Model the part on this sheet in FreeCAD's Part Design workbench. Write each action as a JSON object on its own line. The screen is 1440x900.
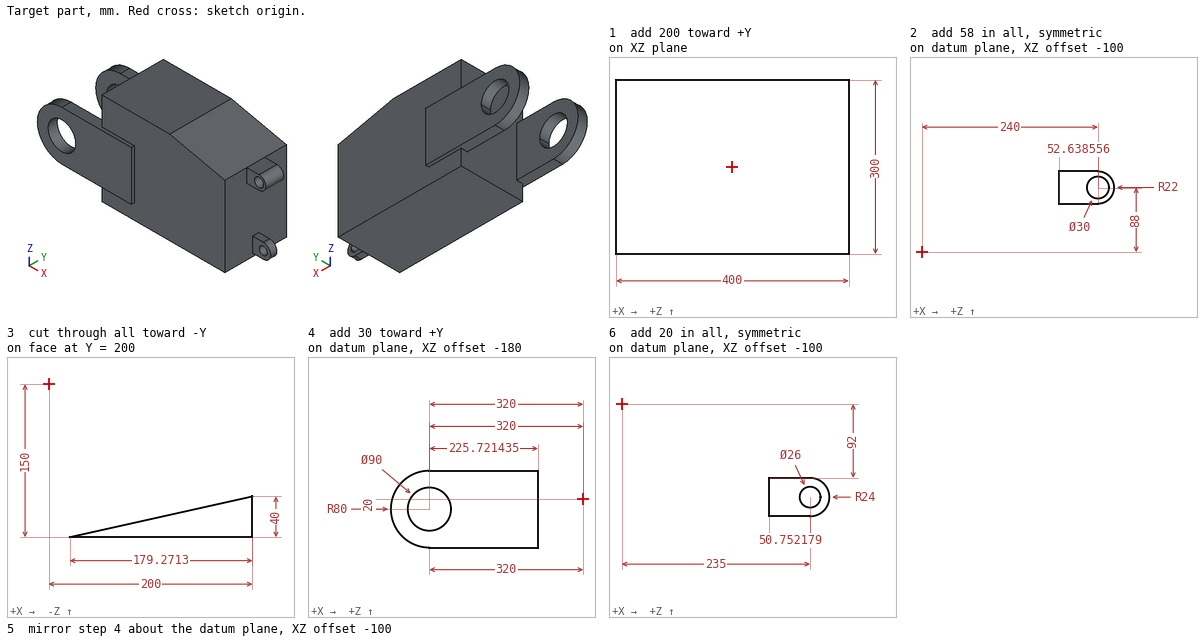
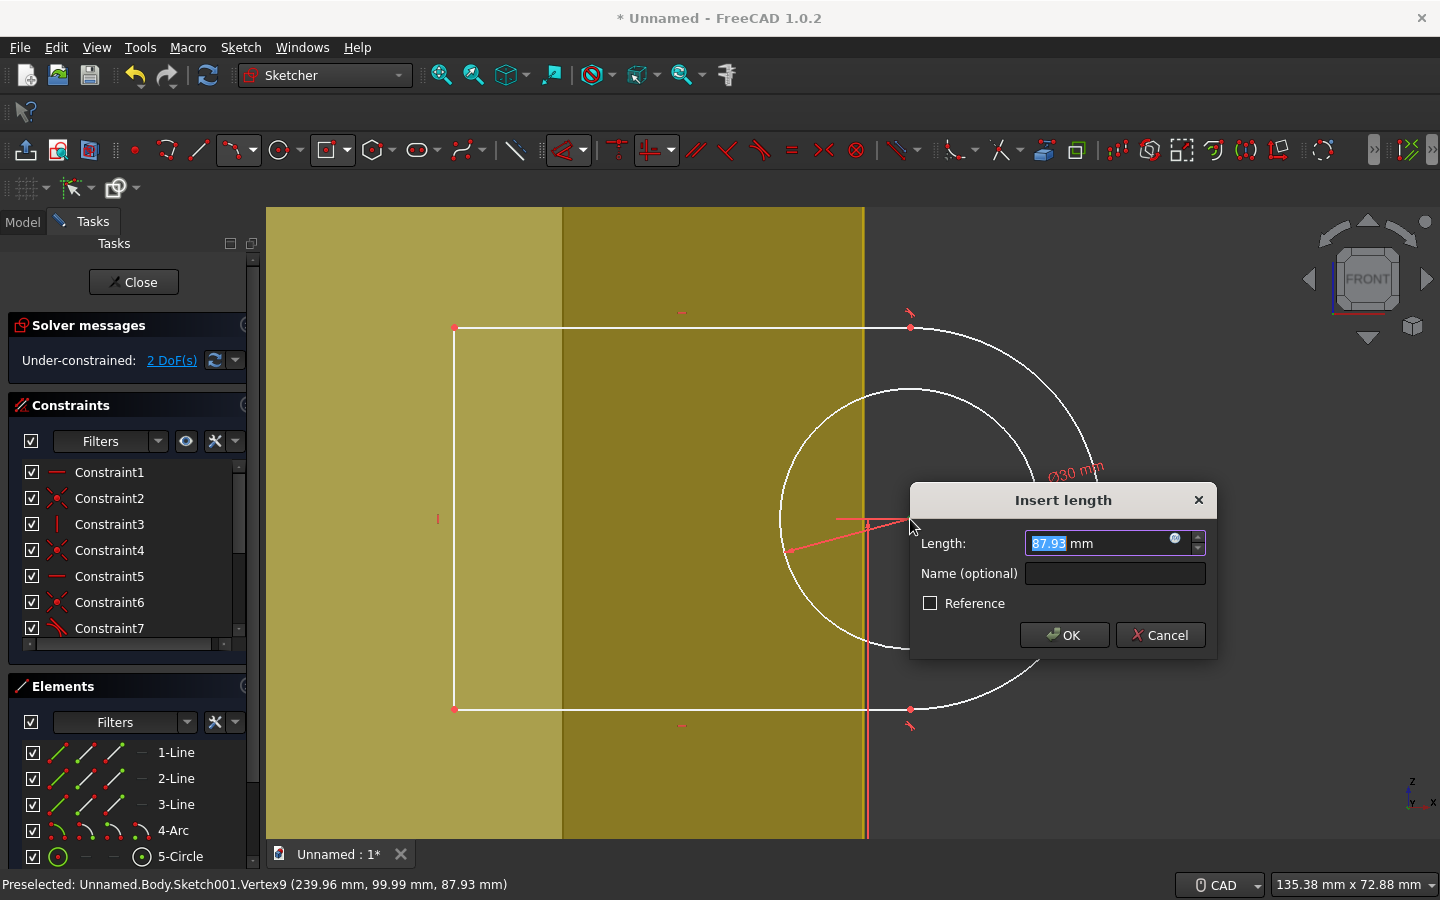
{"action": "type", "text": "88"}
{"action": "key", "text": "Return"}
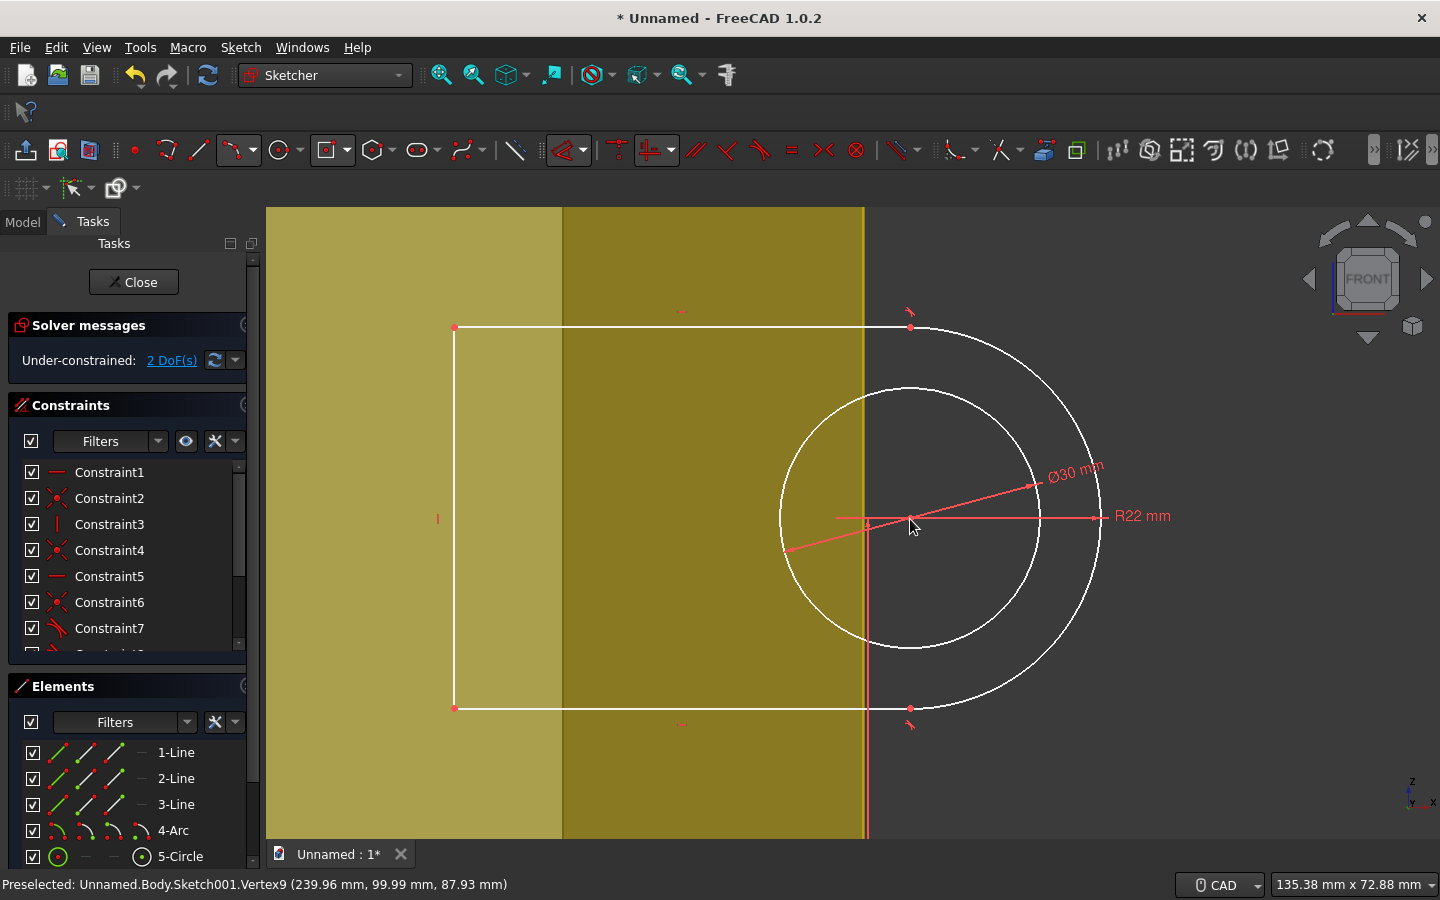
{"action": "left_click", "coordinate": [910, 518]}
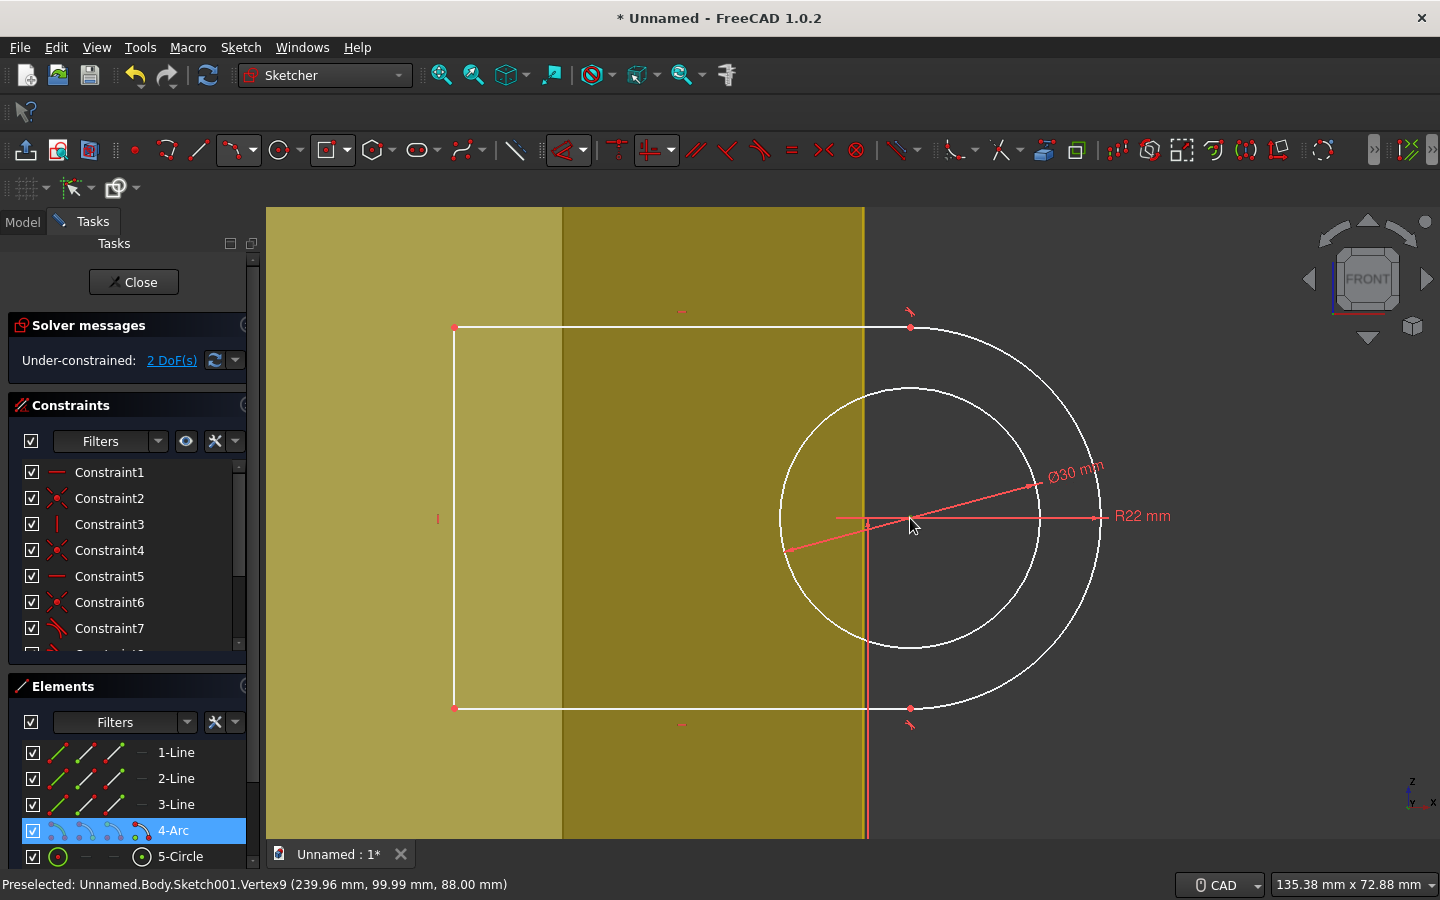
{"action": "left_click", "coordinate": [586, 150]}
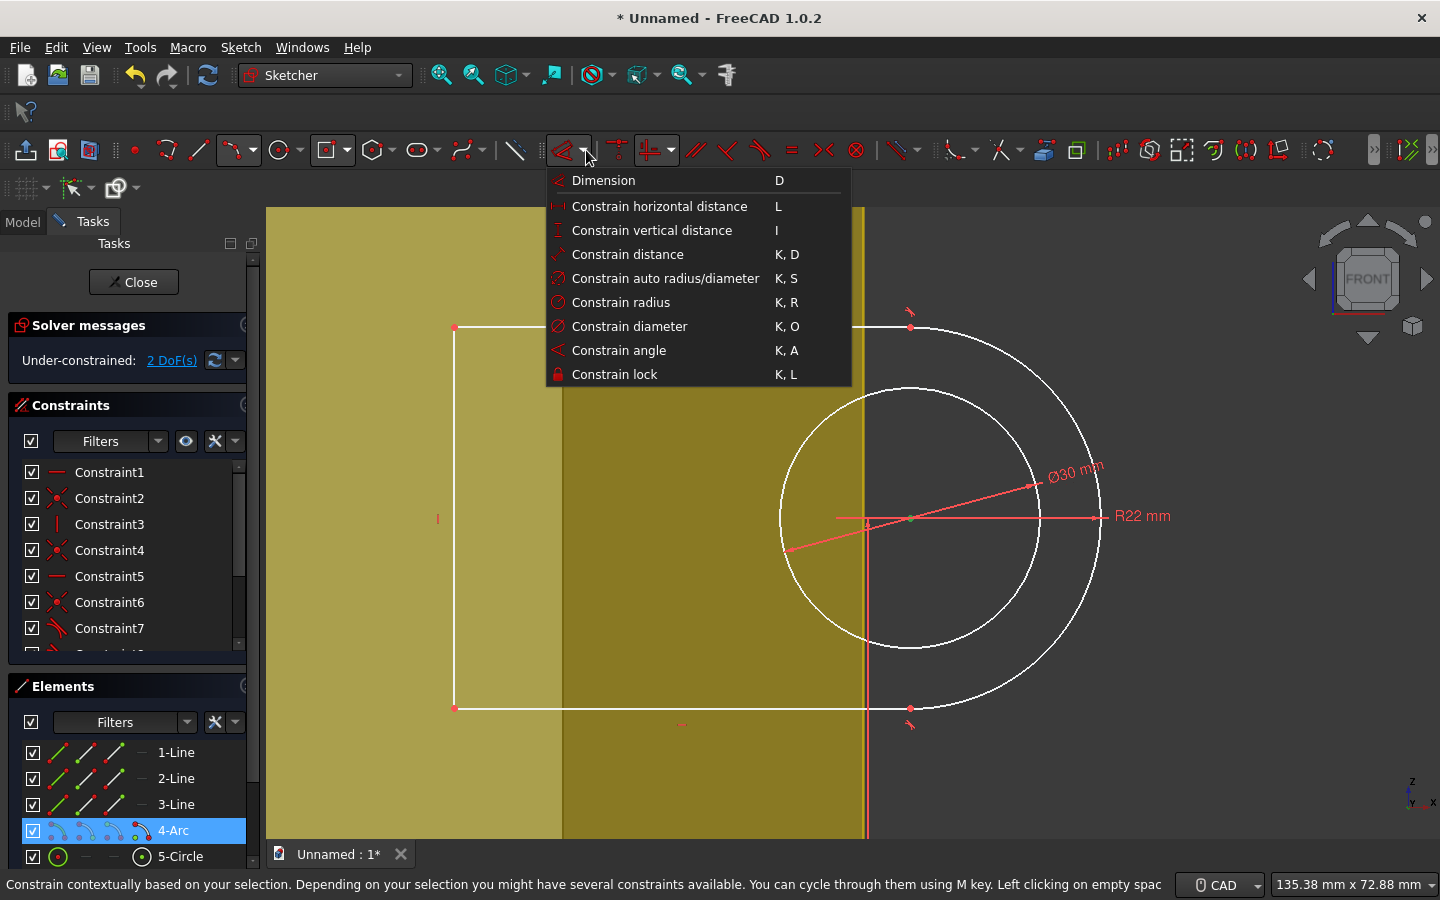
{"action": "left_click", "coordinate": [699, 206]}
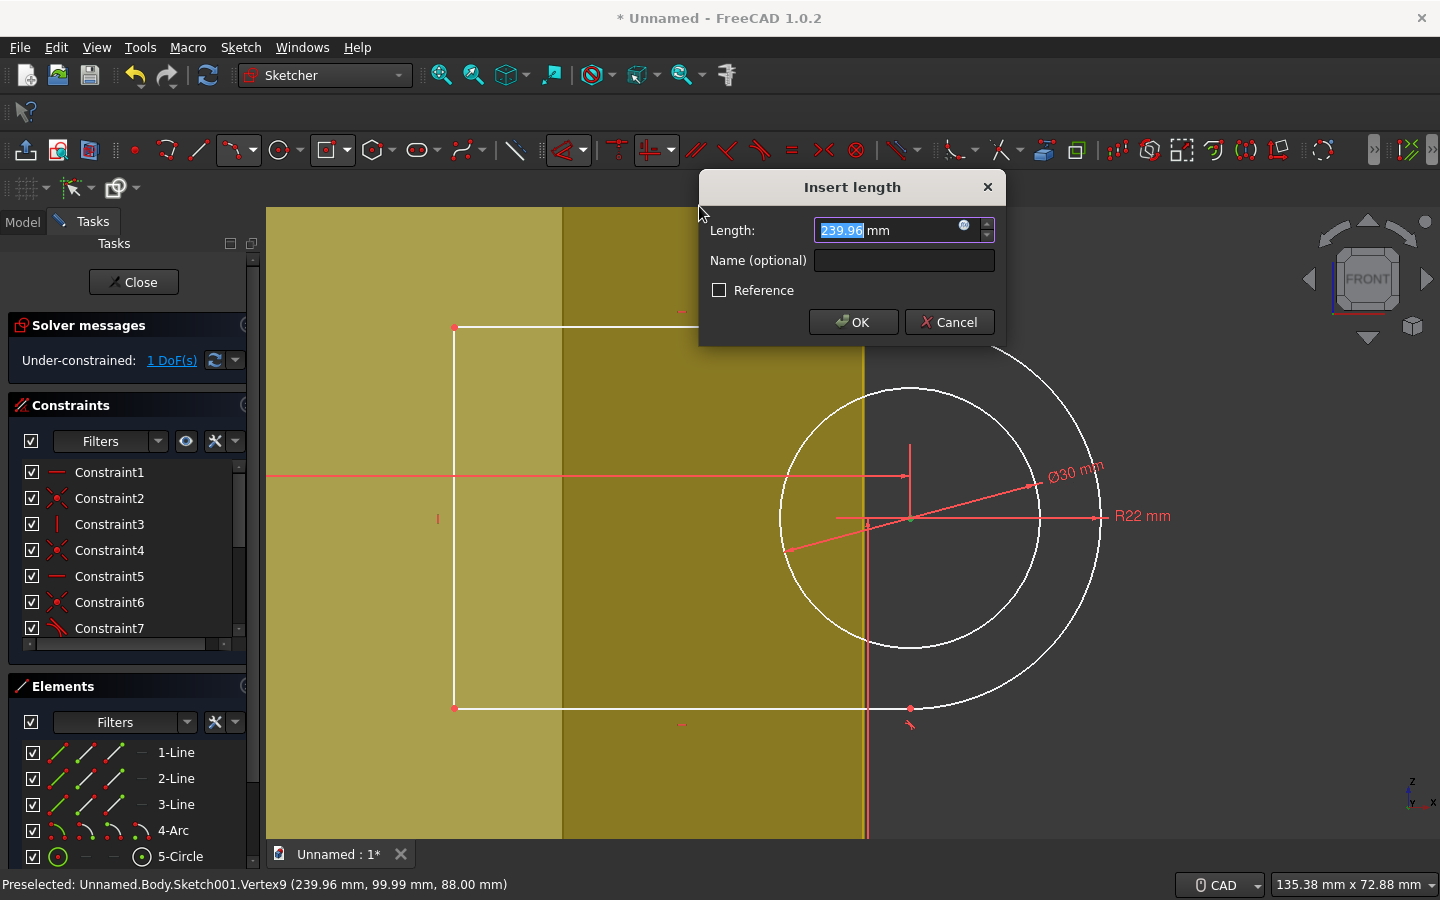
{"action": "type", "text": "240"}
{"action": "key", "text": "Return"}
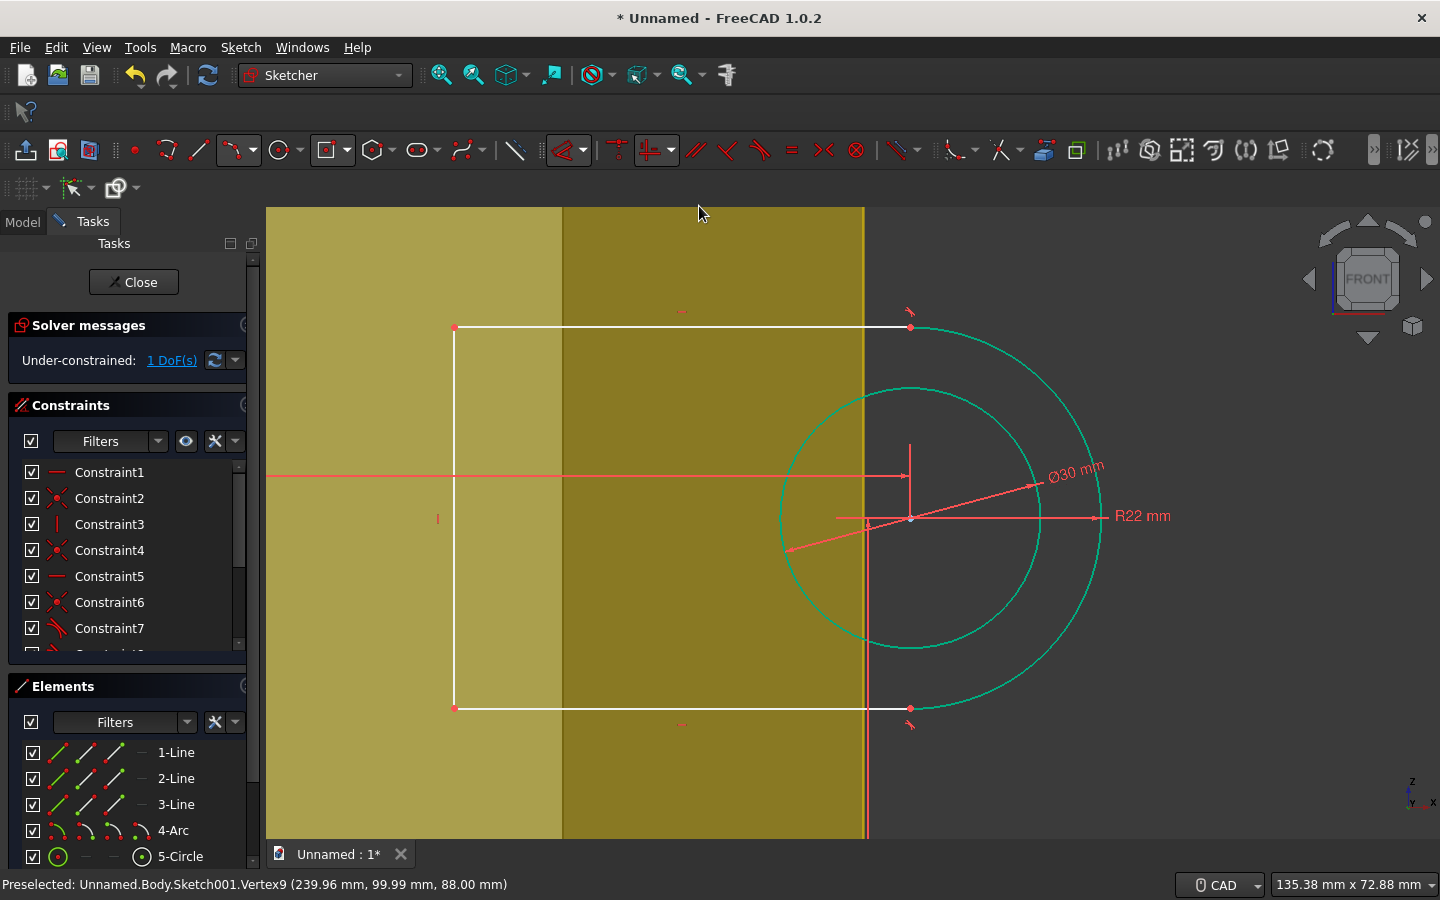
{"action": "left_click", "coordinate": [773, 709]}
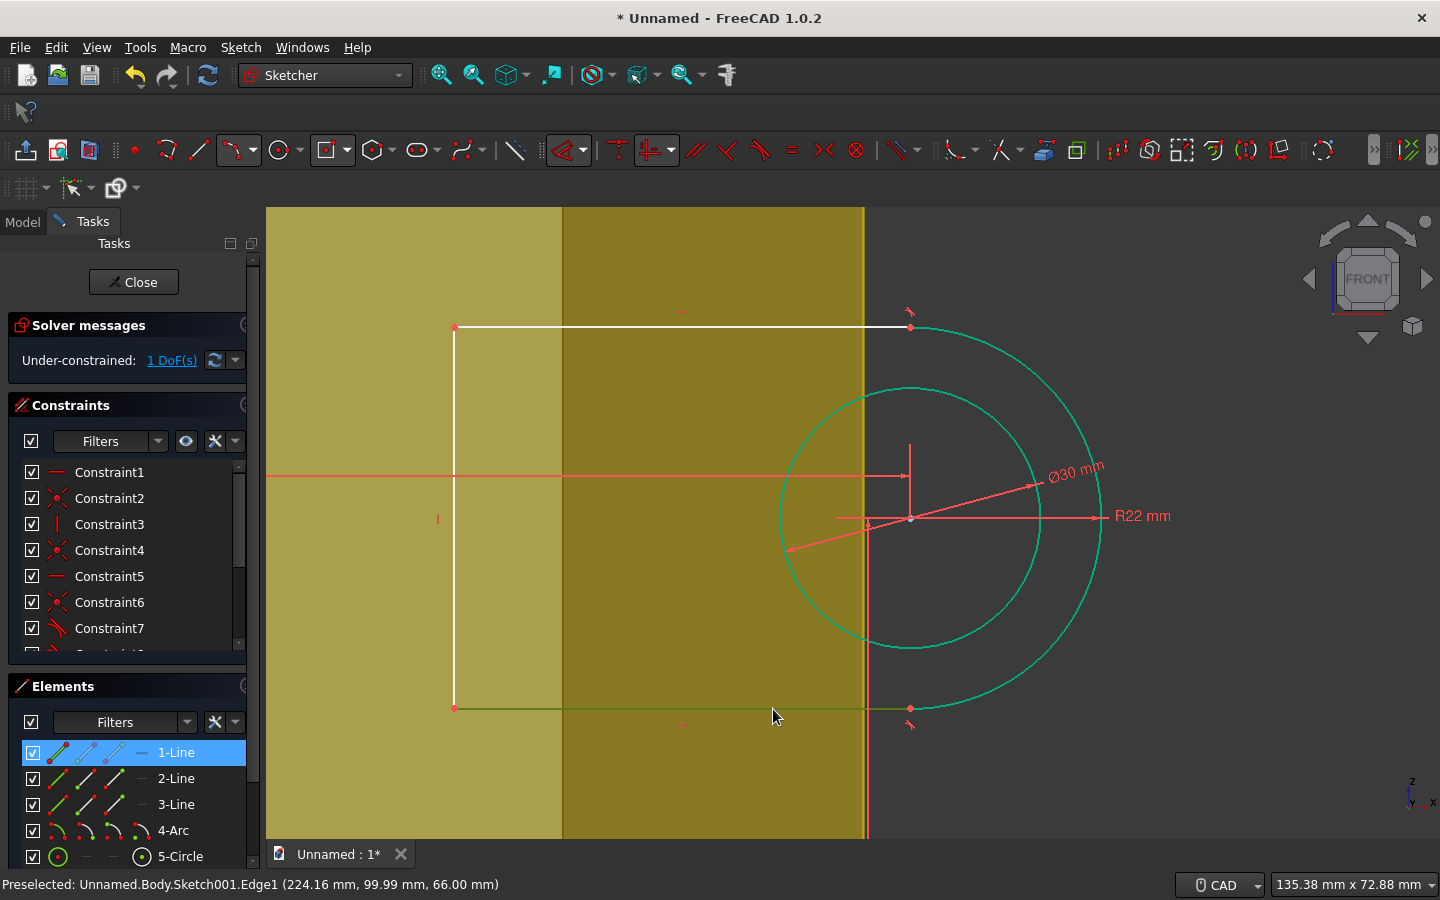
{"action": "key", "text": "l"}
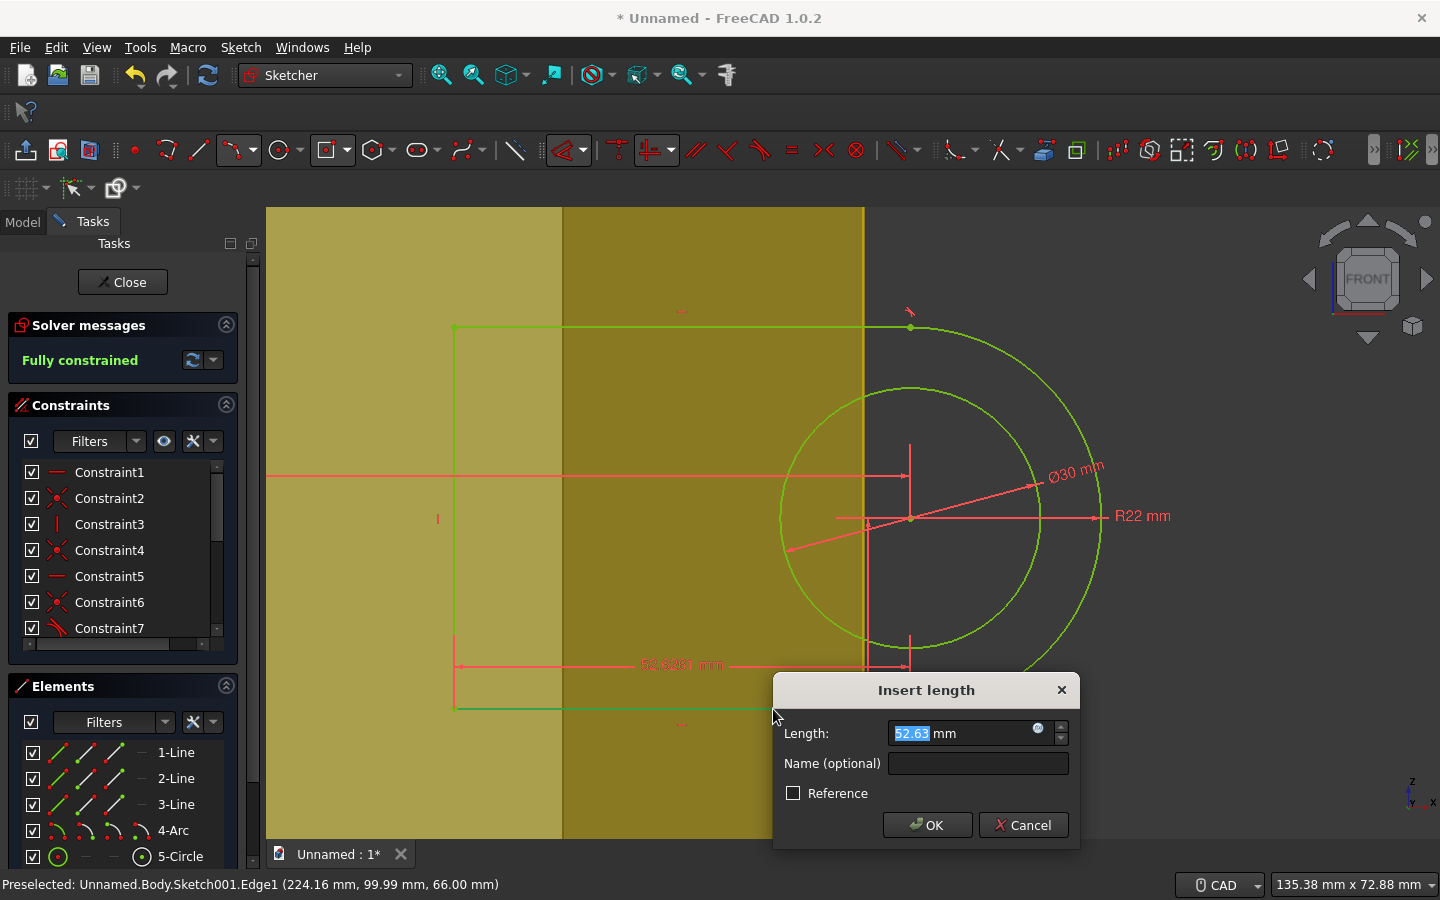
{"action": "type", "text": "52.638556"}
{"action": "key", "text": "Return"}